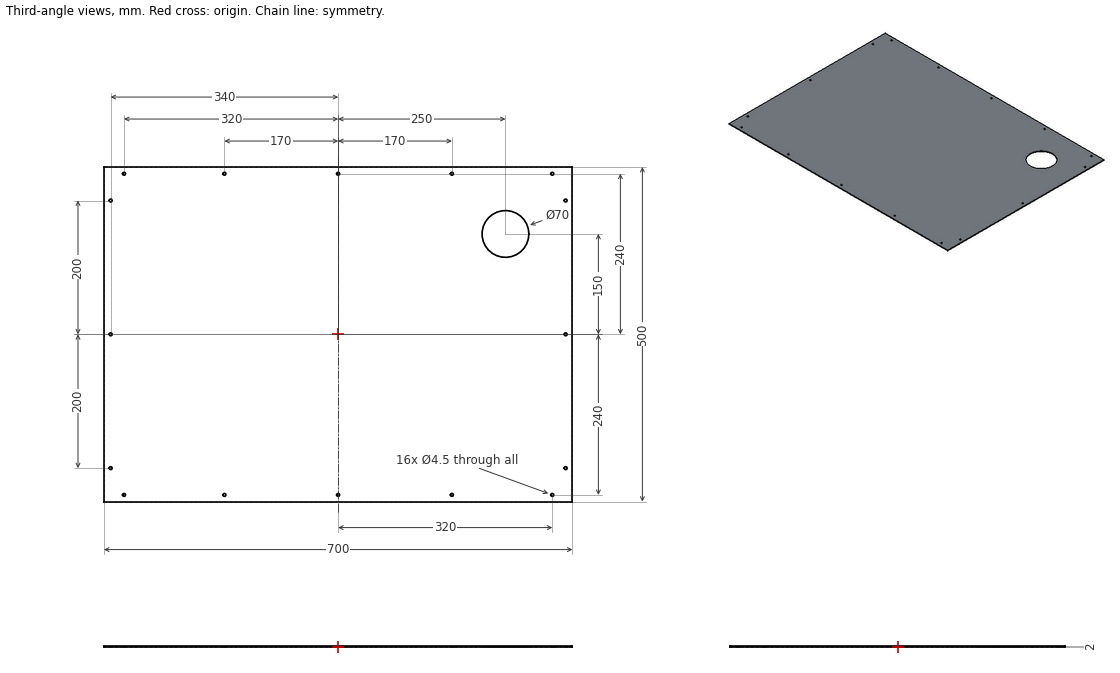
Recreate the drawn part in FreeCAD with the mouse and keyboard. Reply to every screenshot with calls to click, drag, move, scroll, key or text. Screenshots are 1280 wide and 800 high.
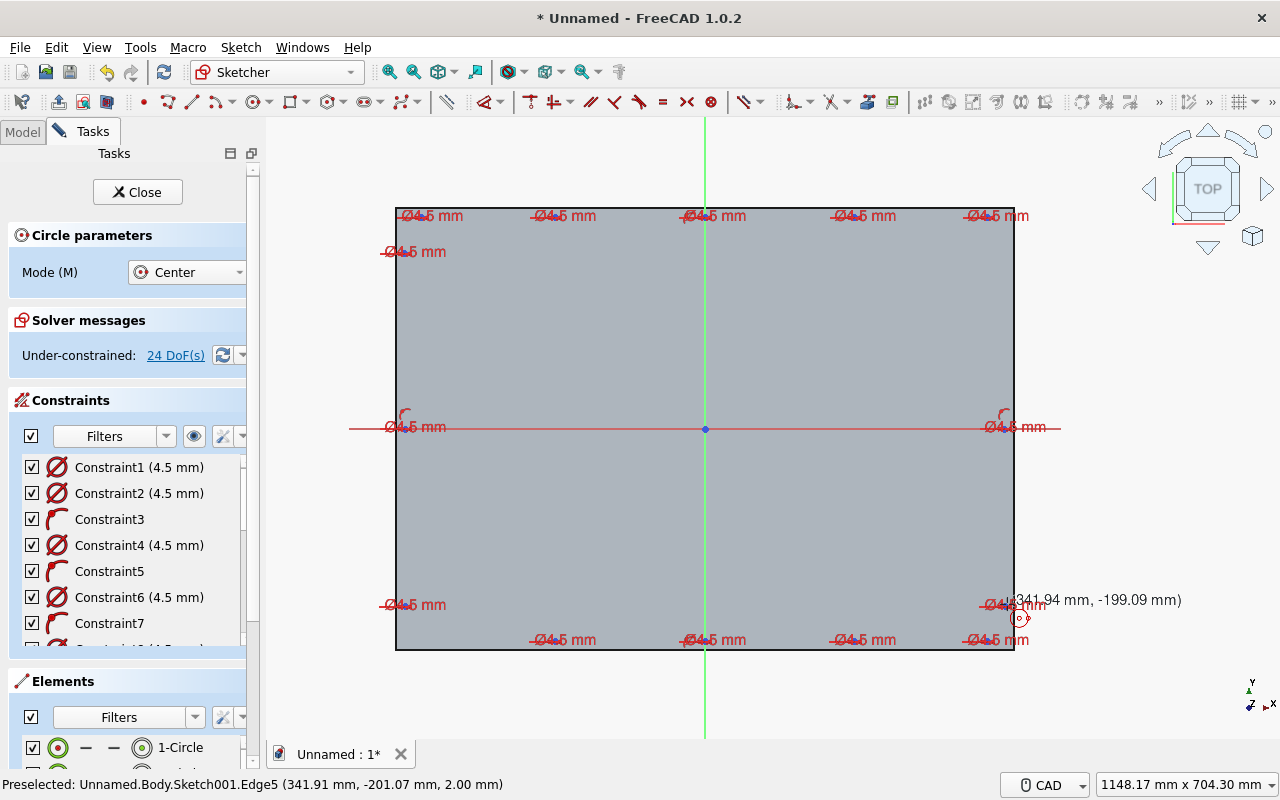
scroll(1005, 253, up, 13)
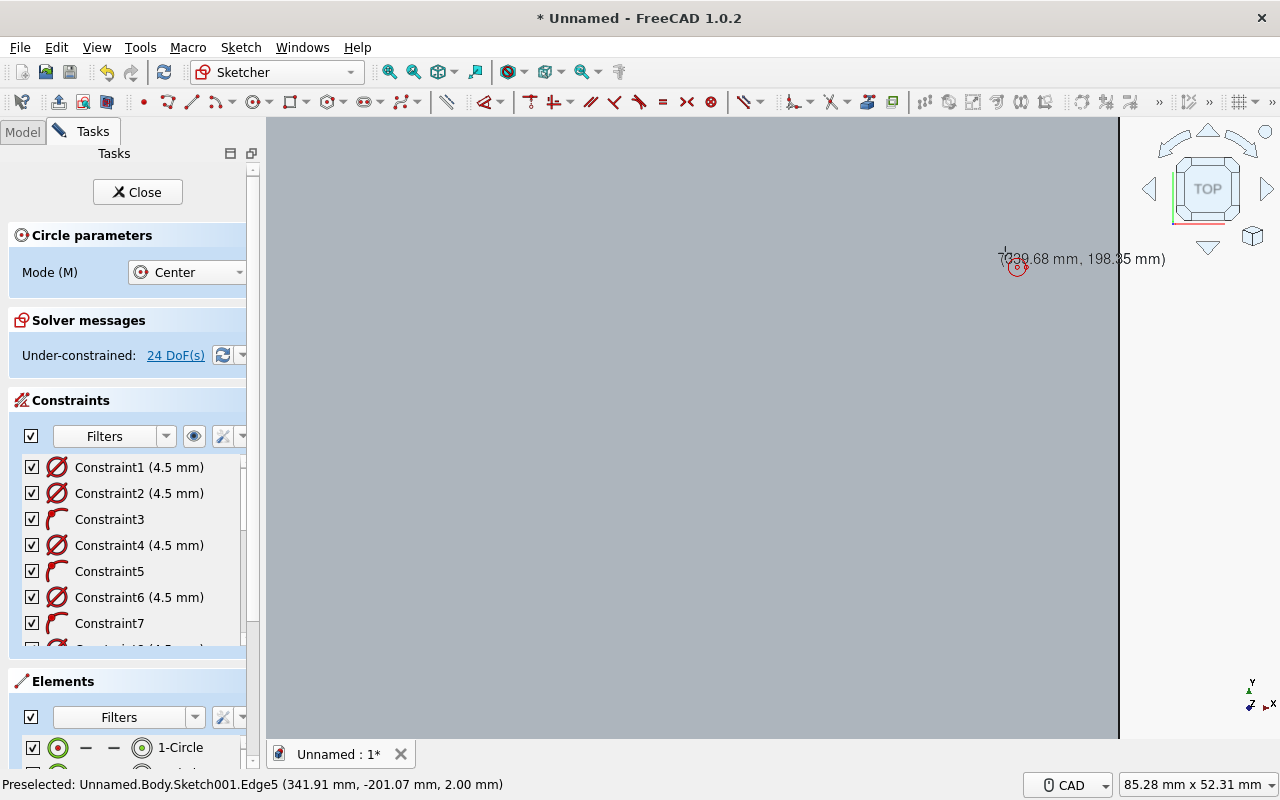
scroll(1005, 252, down, 13)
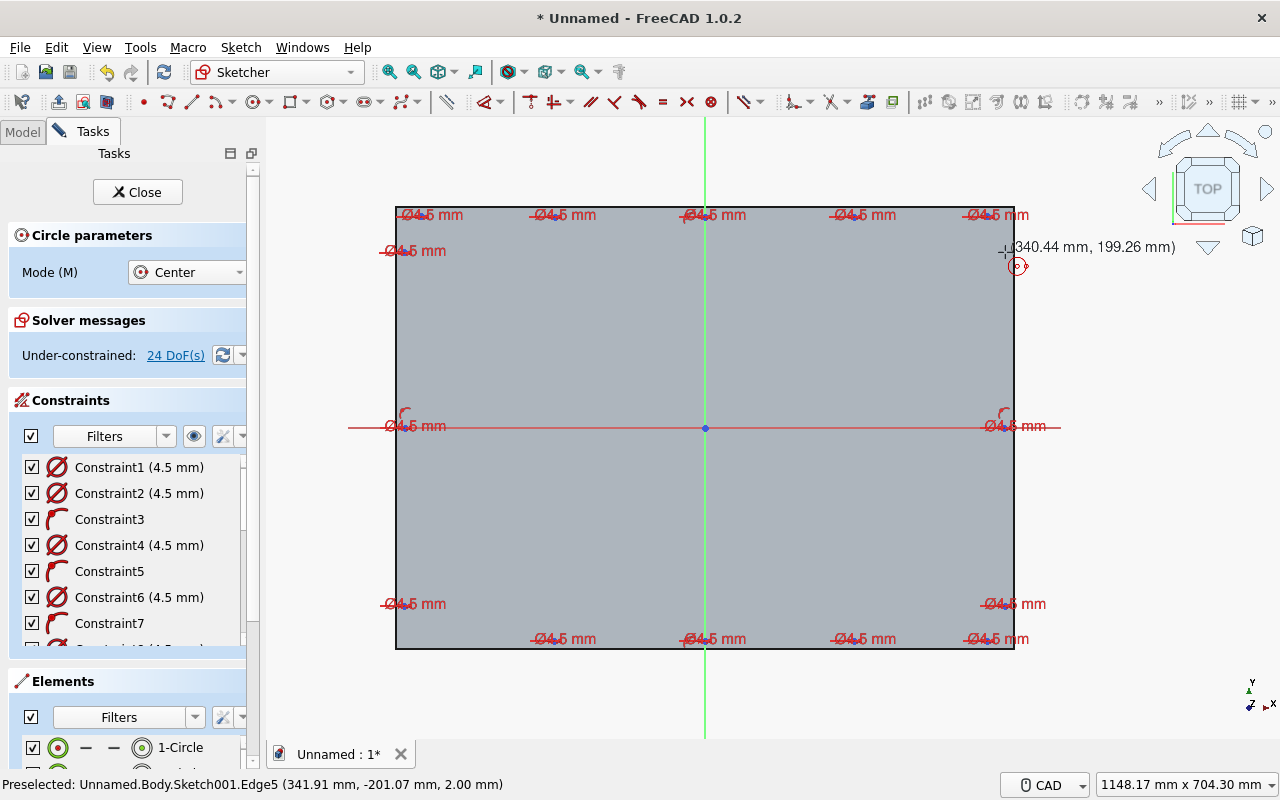
click(1005, 252)
move(1007, 250)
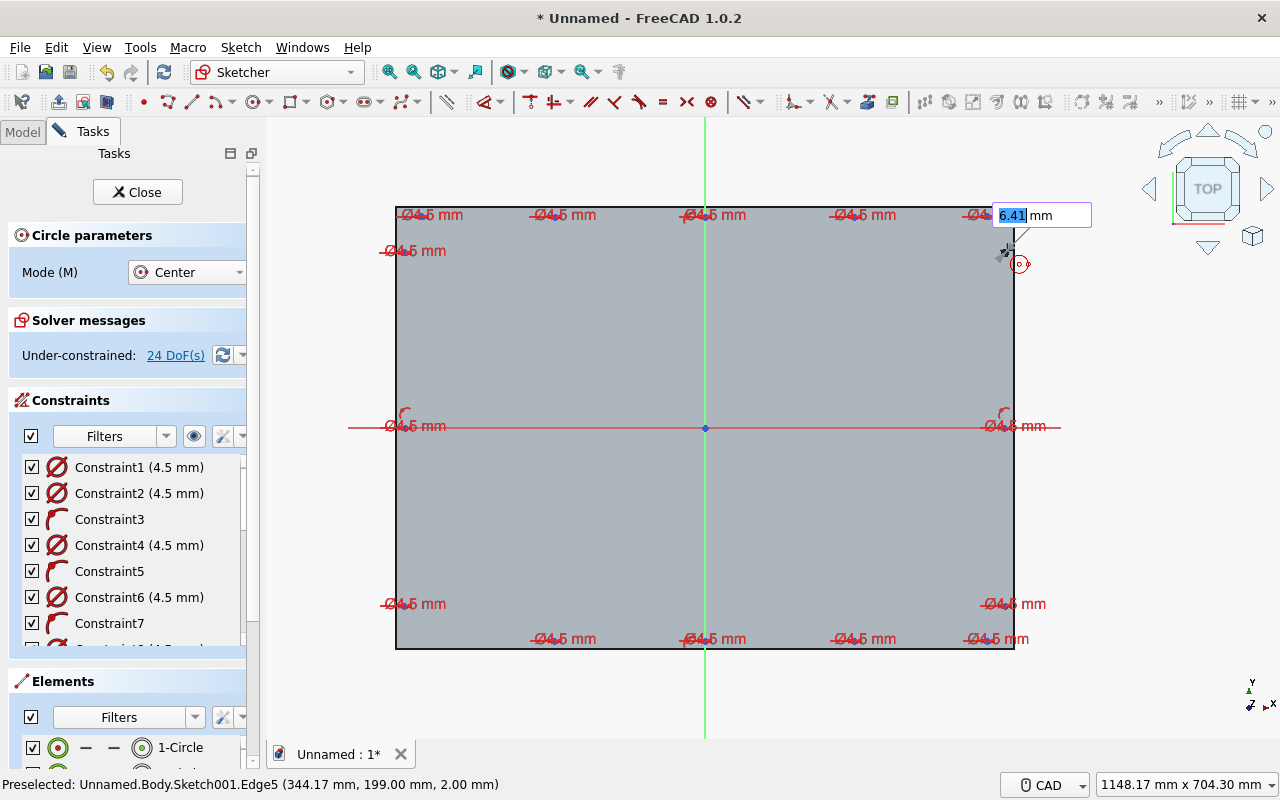
text(4.5)
key(Return)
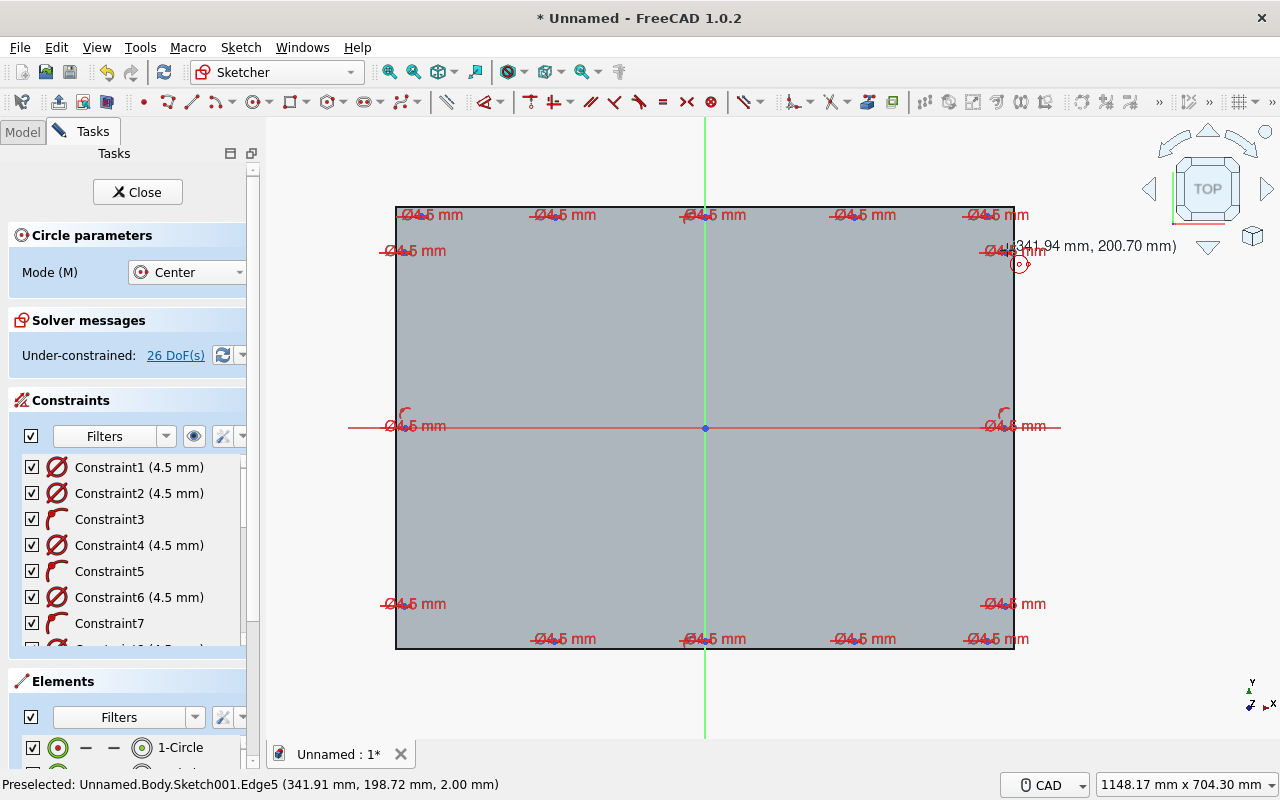
scroll(422, 640, up, 13)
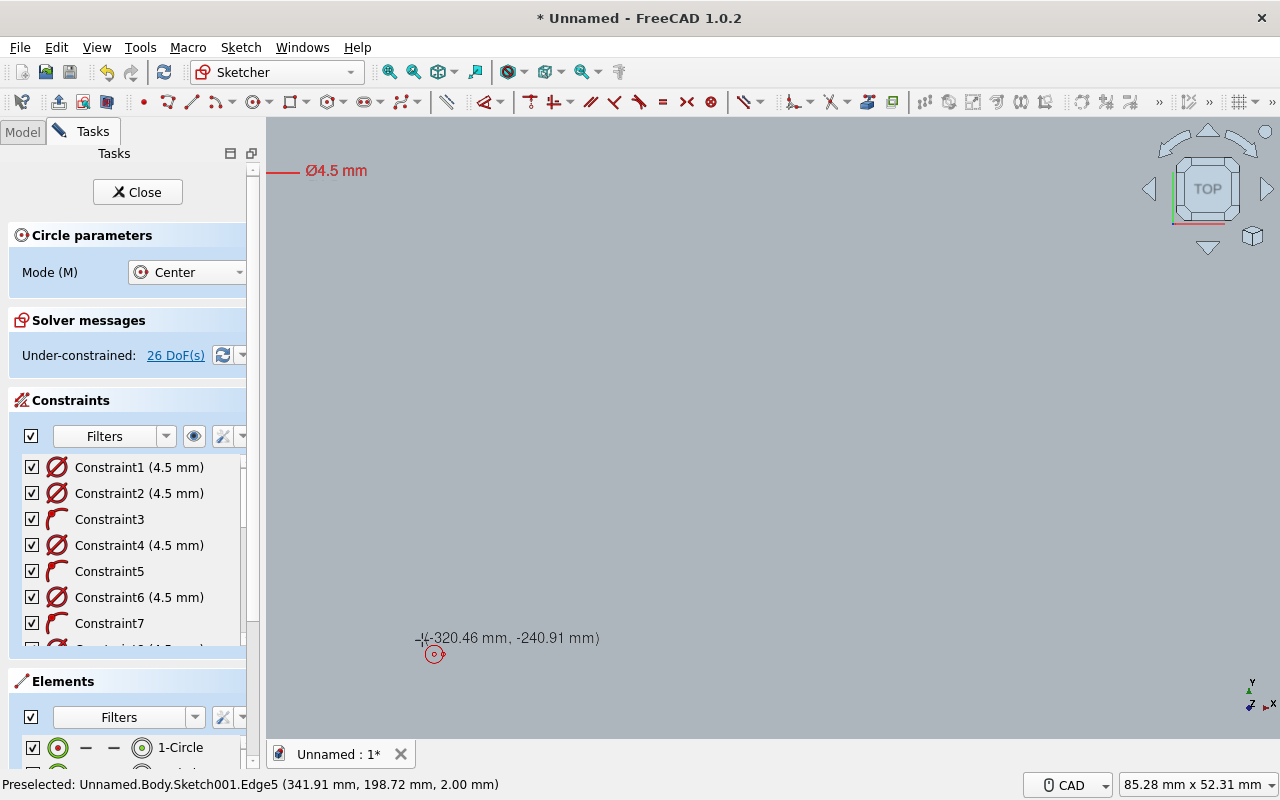
scroll(422, 641, down, 13)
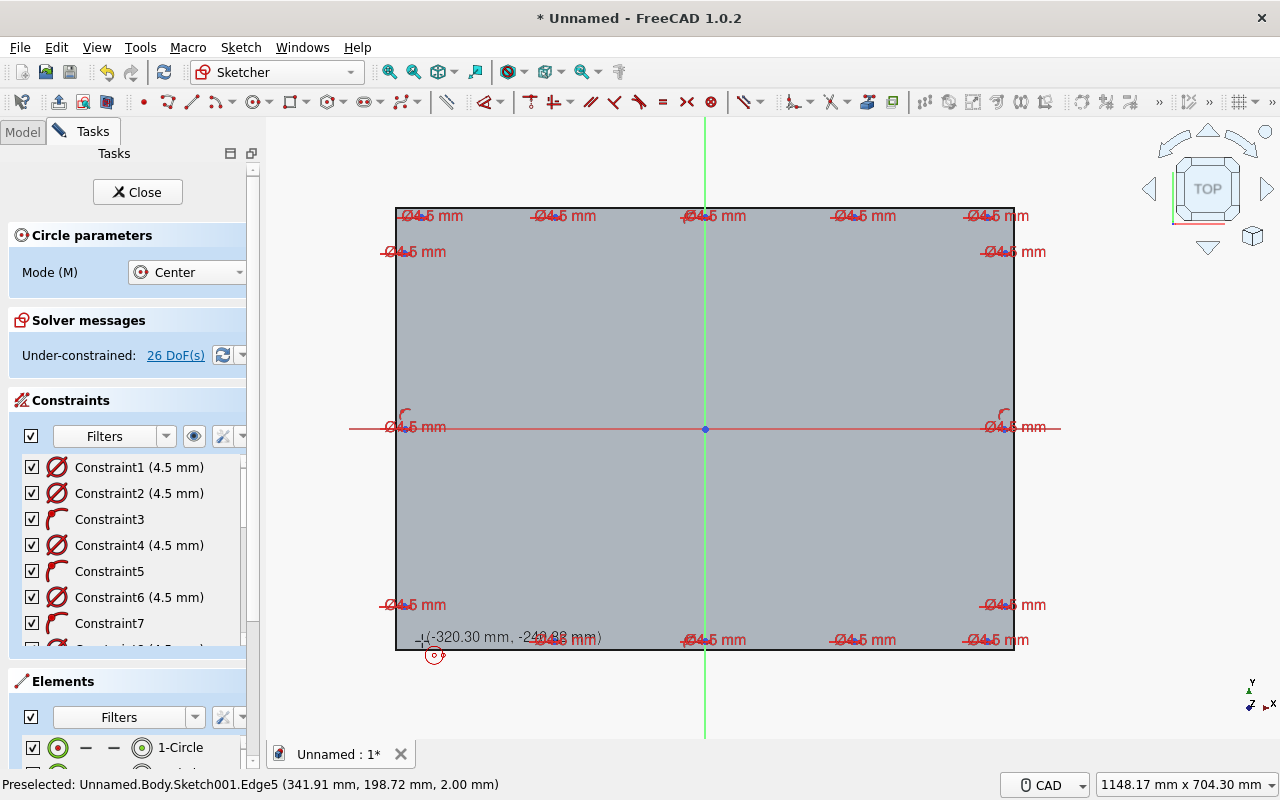
click(422, 641)
move(424, 640)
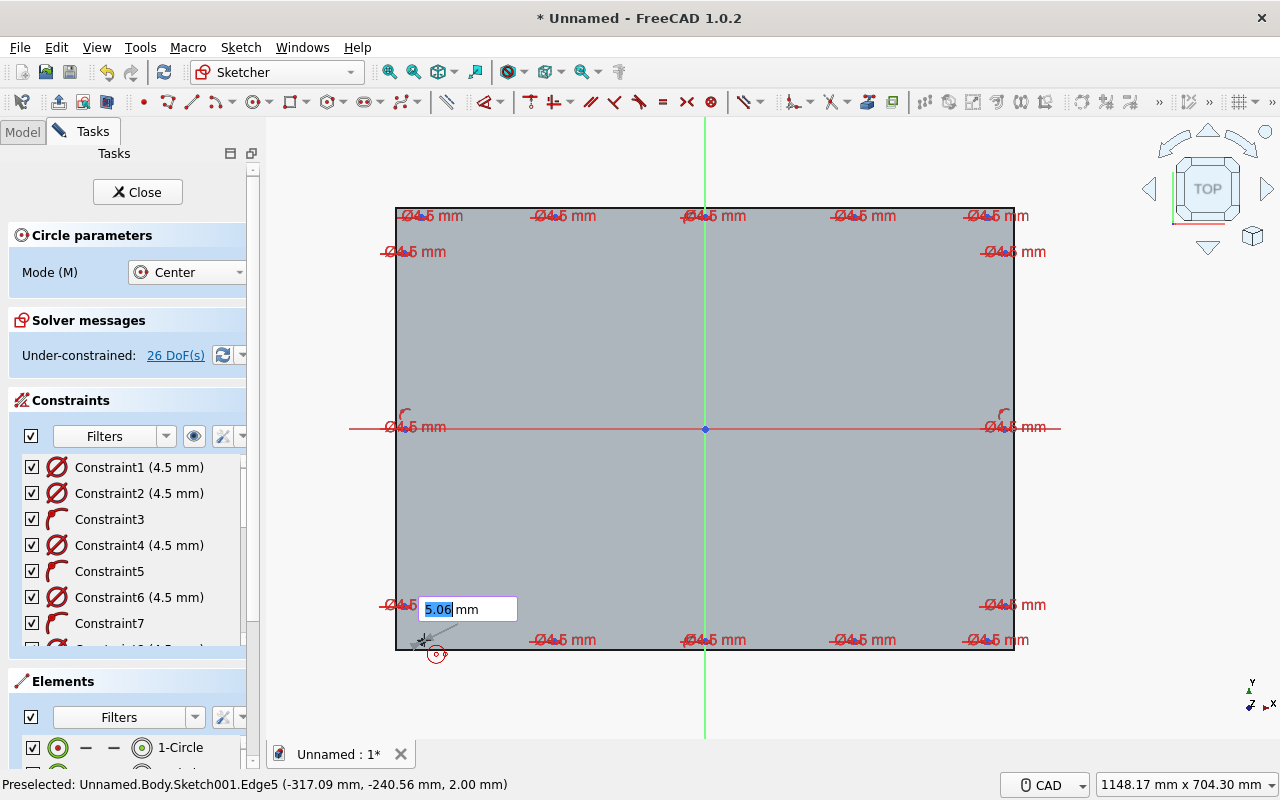
text(4.5)
key(Return)
key(Escape)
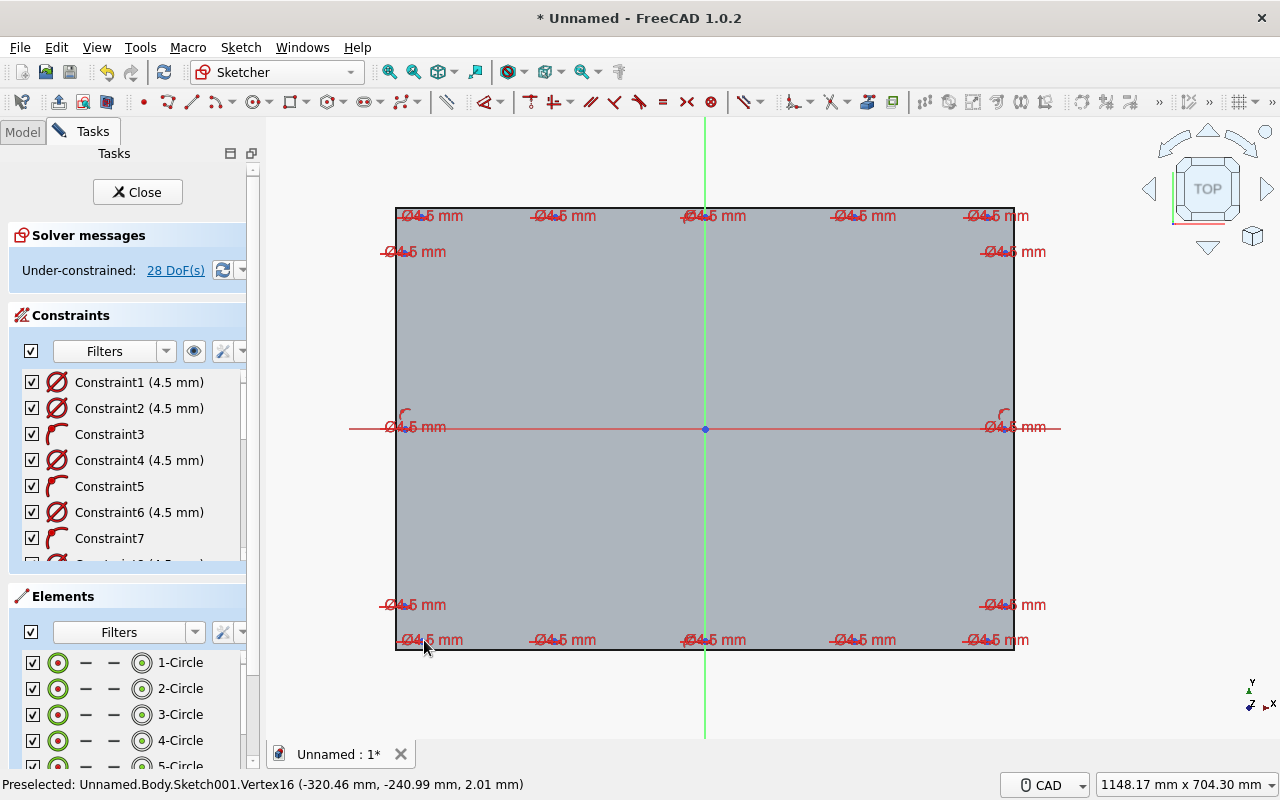
click(988, 642)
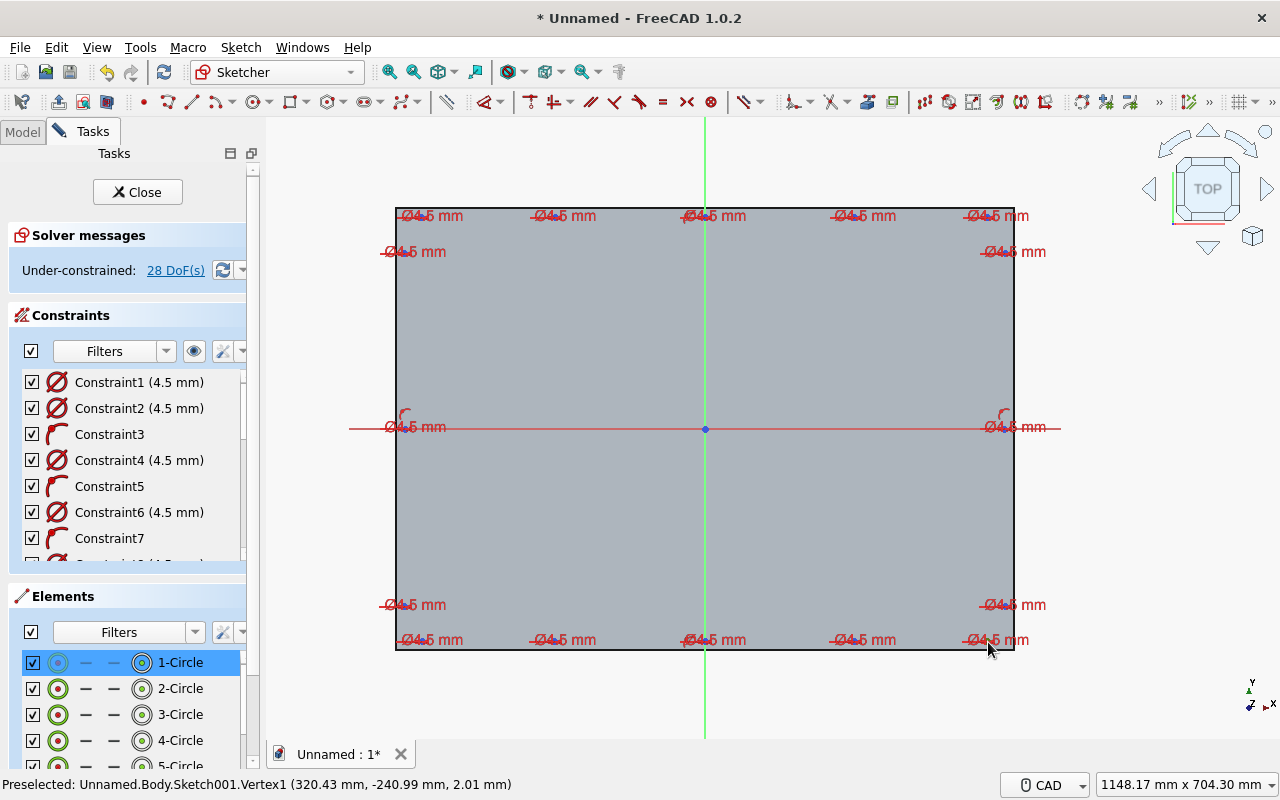
click(705, 642)